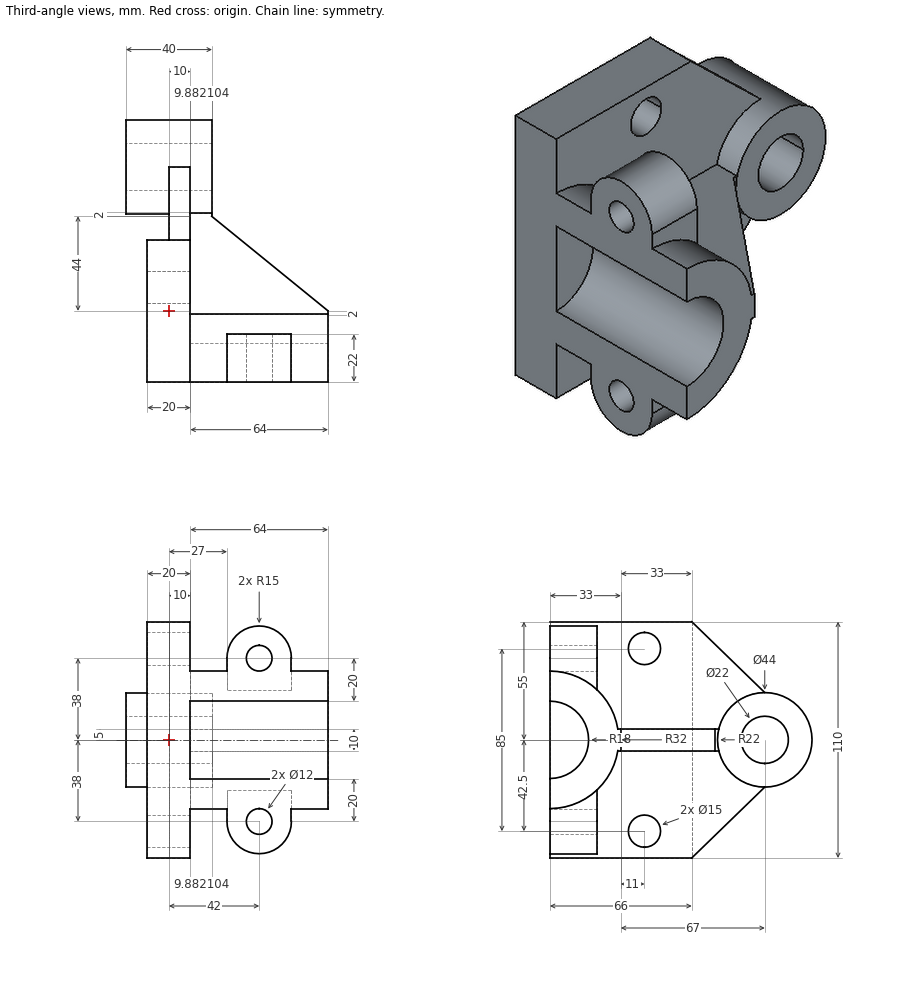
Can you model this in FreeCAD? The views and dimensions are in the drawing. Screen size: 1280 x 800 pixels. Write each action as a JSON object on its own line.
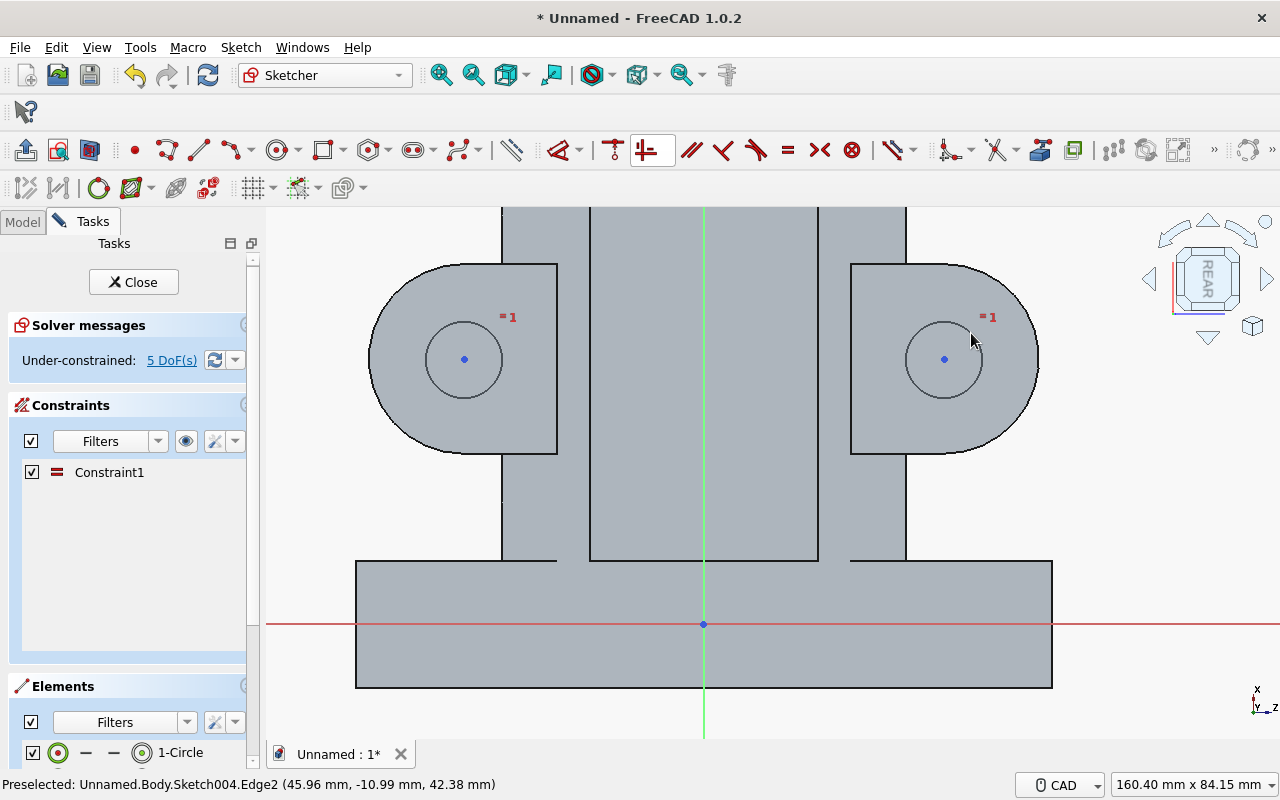
{"action": "left_click", "coordinate": [464, 360]}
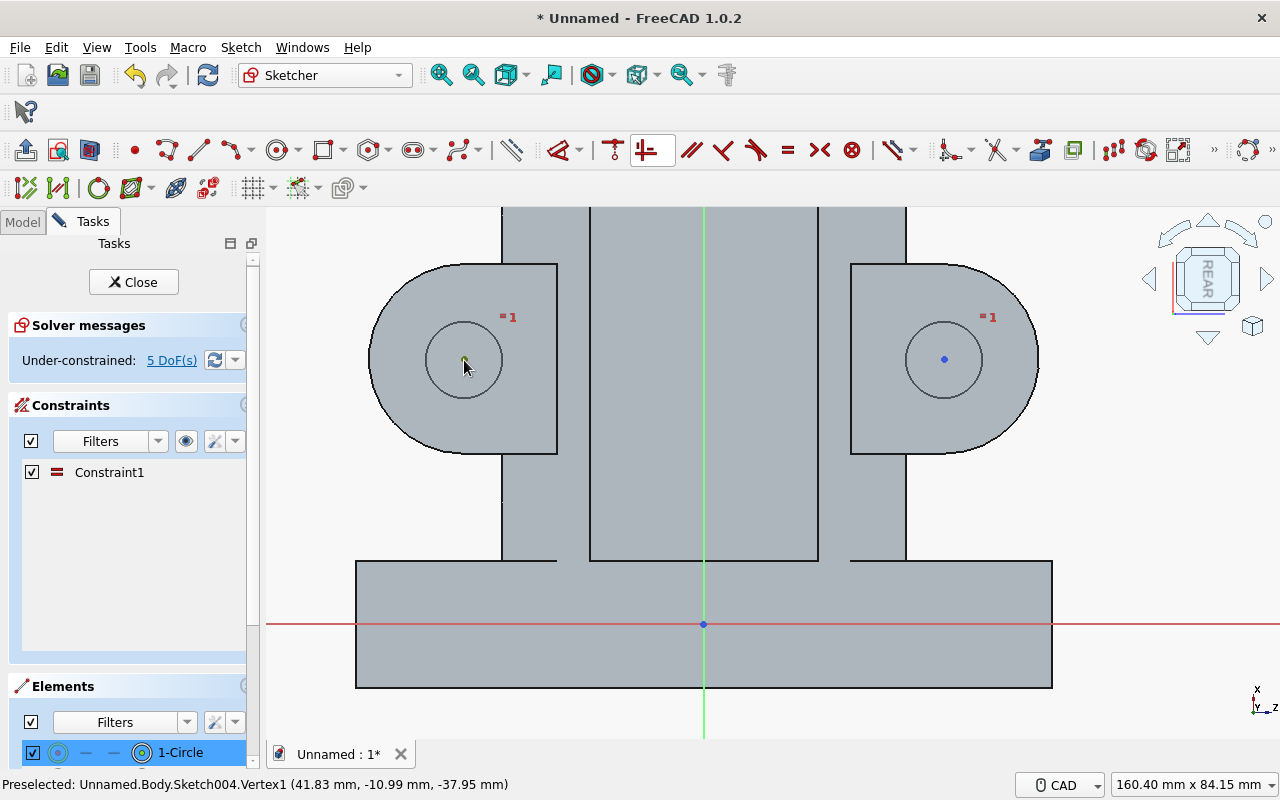
{"action": "left_click", "coordinate": [944, 360]}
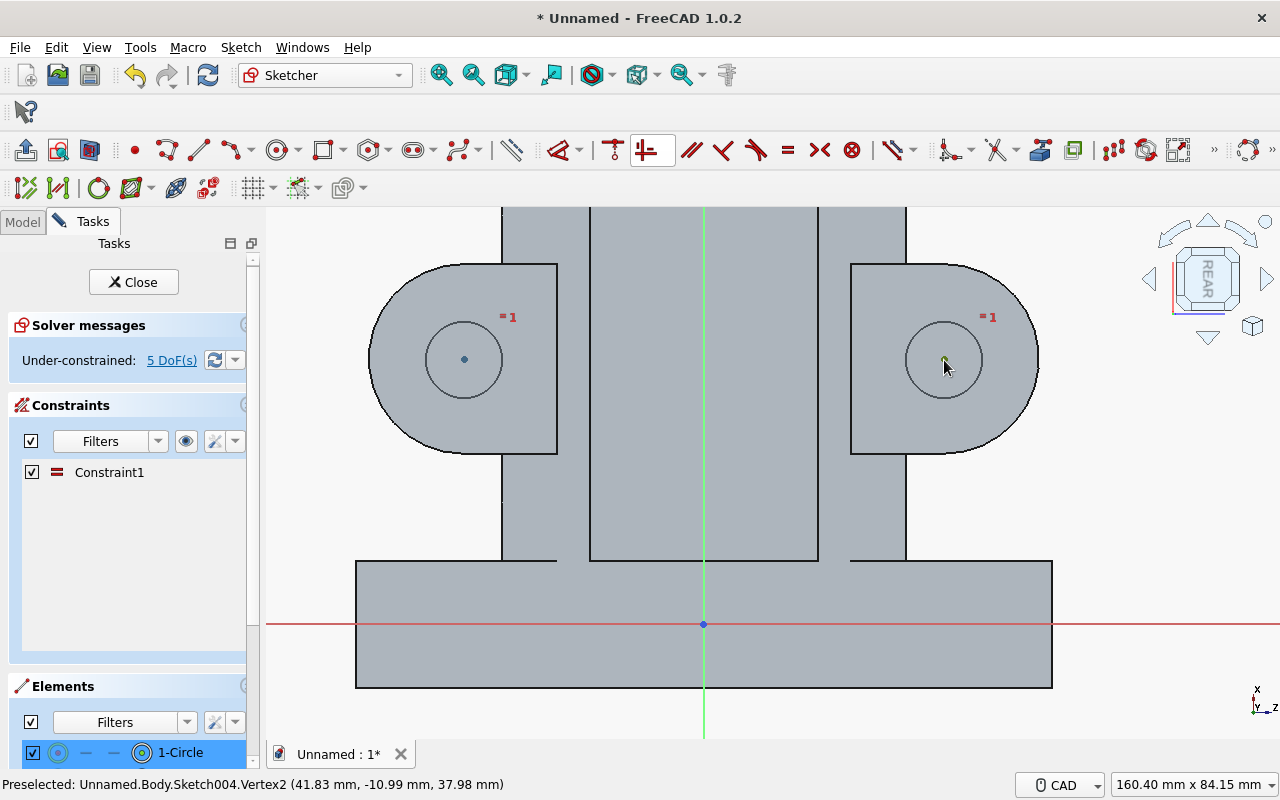
{"action": "left_click", "coordinate": [670, 150]}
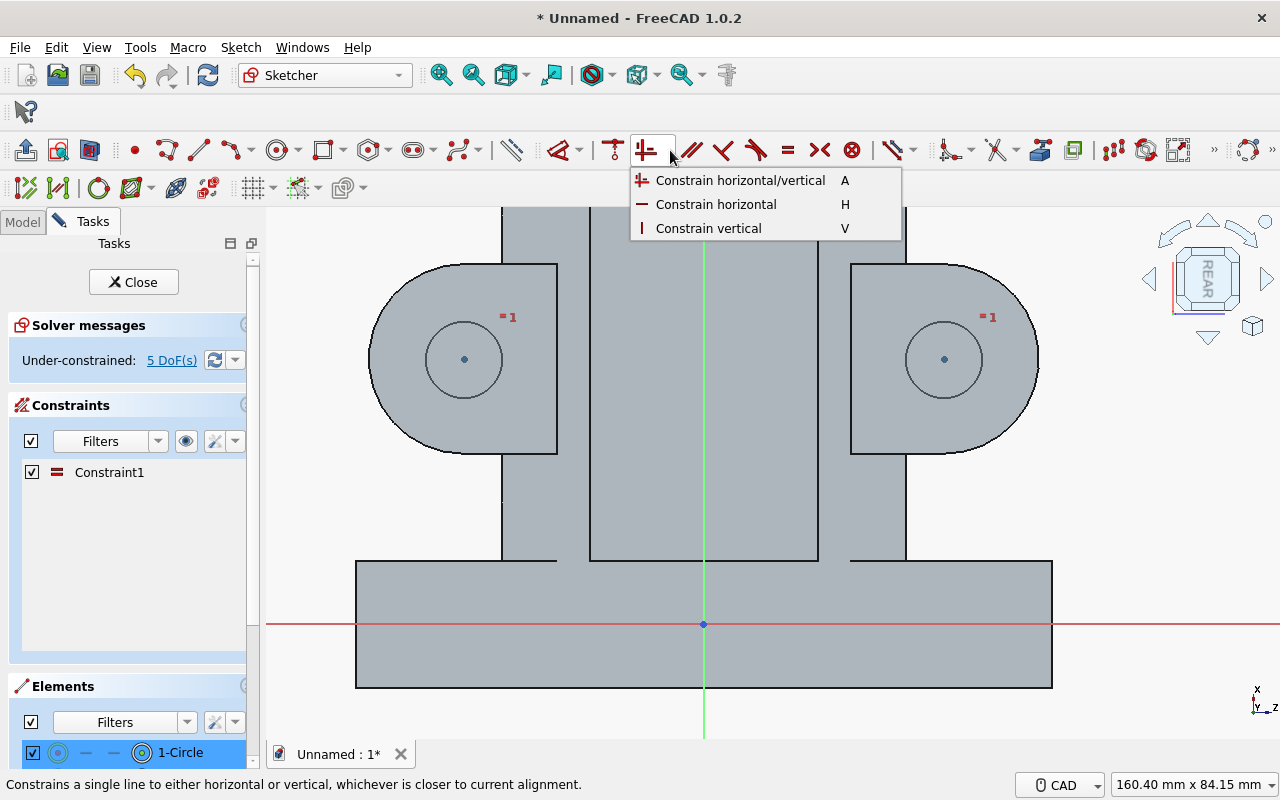
{"action": "left_click", "coordinate": [766, 204]}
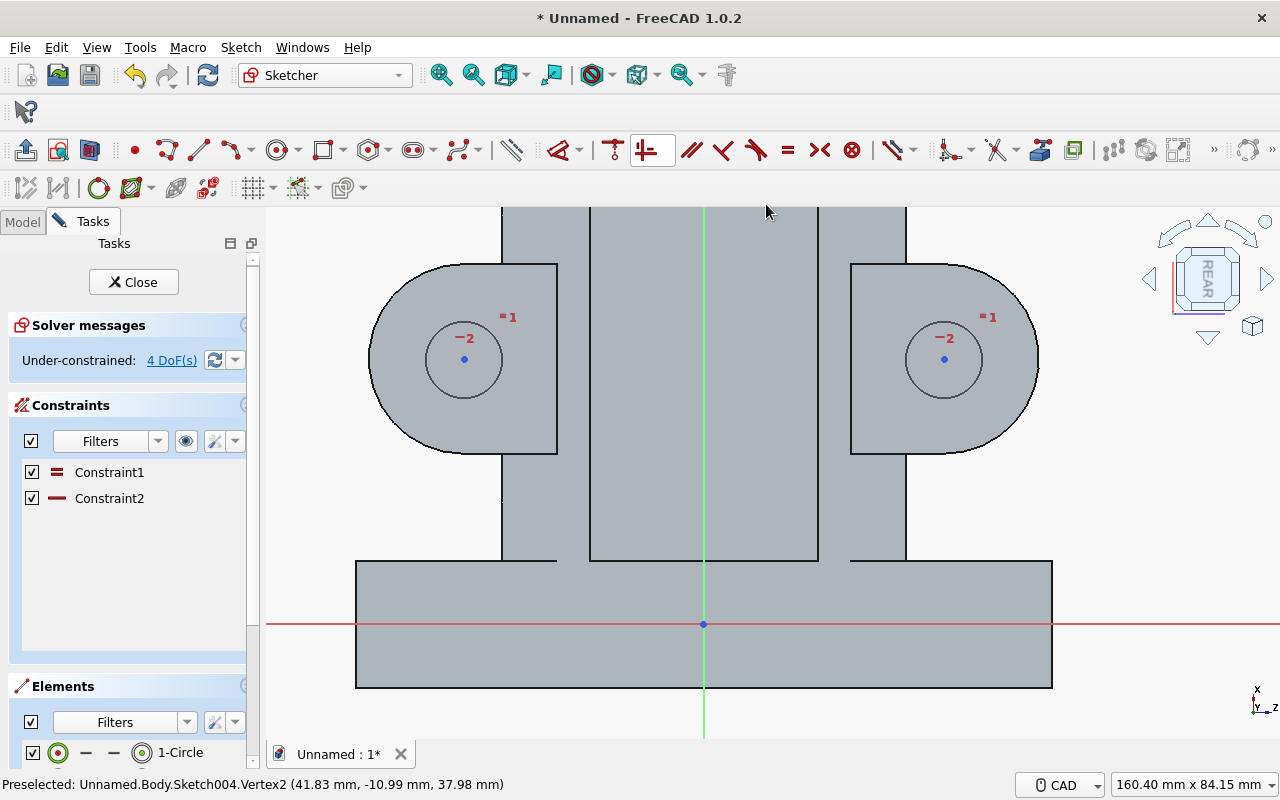
{"action": "left_click", "coordinate": [558, 150]}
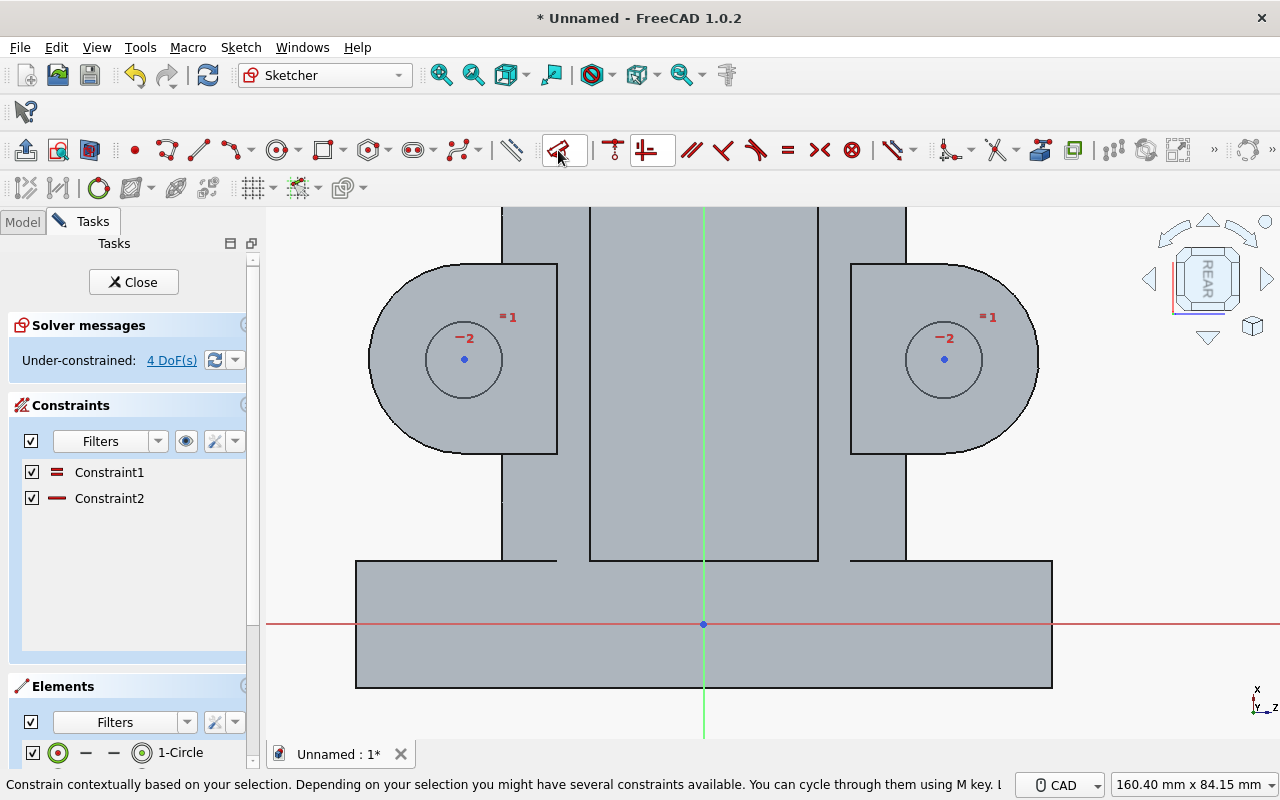
{"action": "left_click", "coordinate": [491, 333]}
{"action": "left_click", "coordinate": [514, 310]}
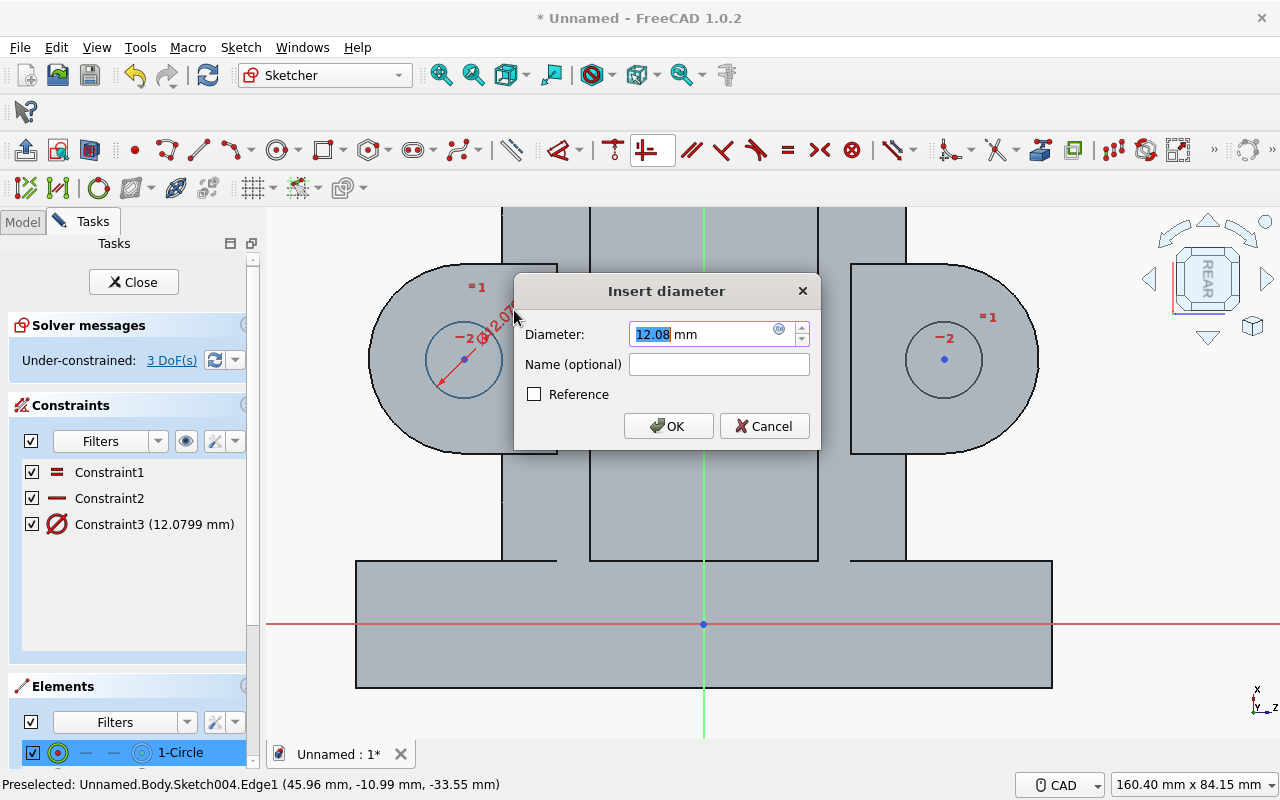
{"action": "type", "text": "12"}
{"action": "key", "text": "Return"}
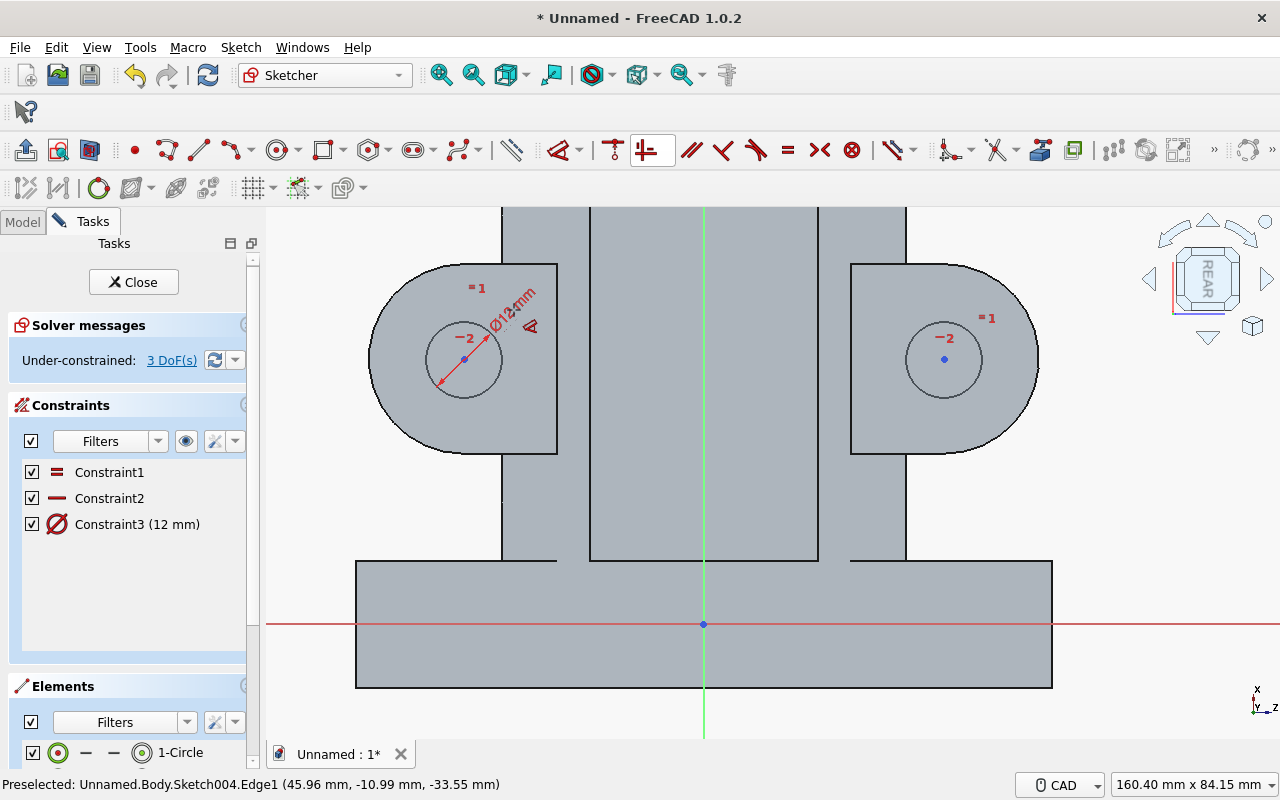
{"action": "left_click", "coordinate": [464, 360]}
{"action": "left_click", "coordinate": [584, 658]}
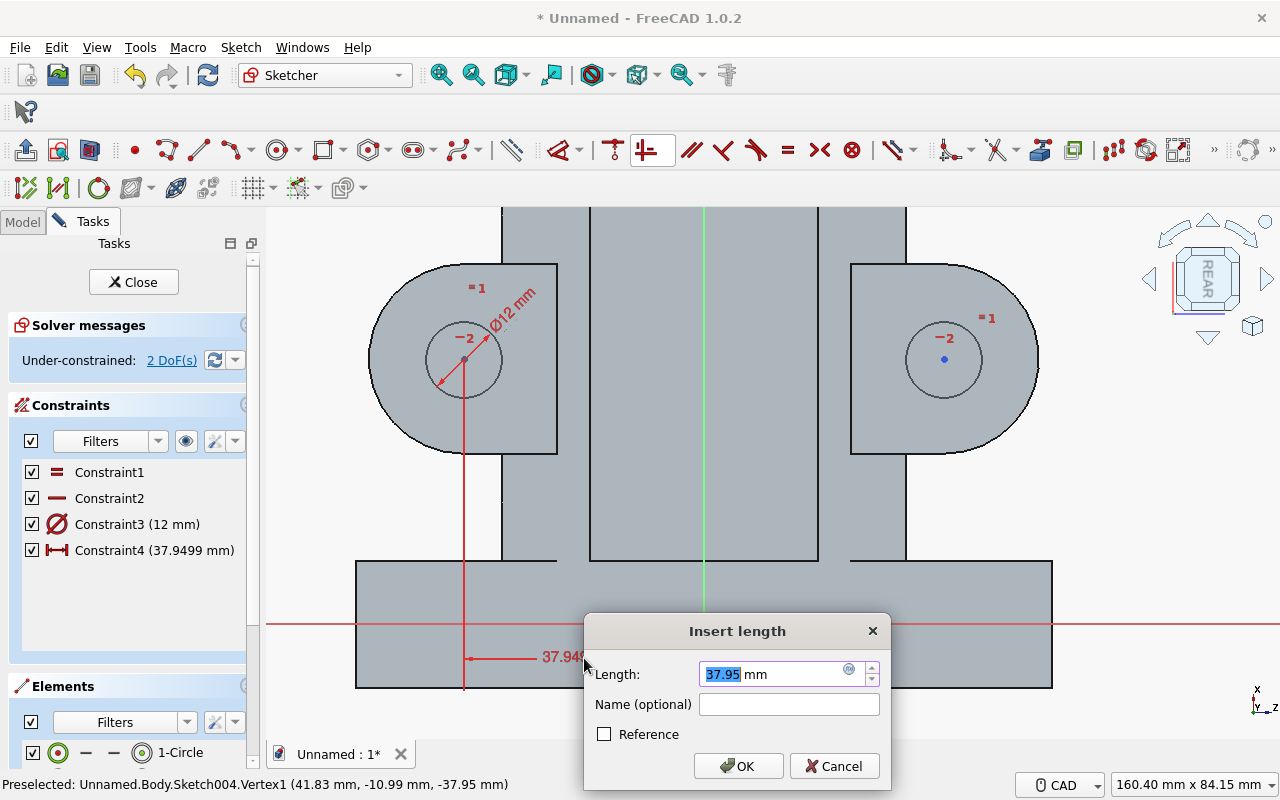
{"action": "type", "text": "38"}
{"action": "key", "text": "Return"}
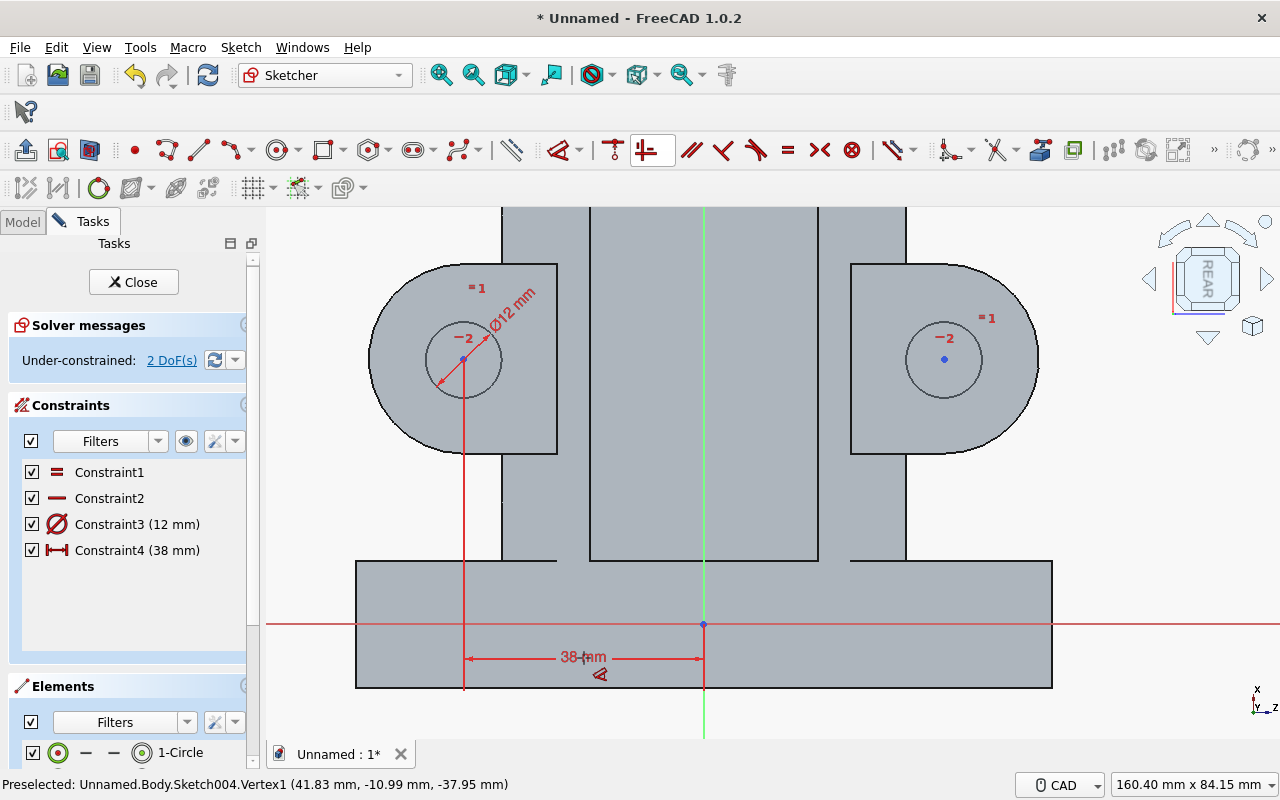
{"action": "left_click", "coordinate": [464, 360]}
{"action": "left_click", "coordinate": [430, 492]}